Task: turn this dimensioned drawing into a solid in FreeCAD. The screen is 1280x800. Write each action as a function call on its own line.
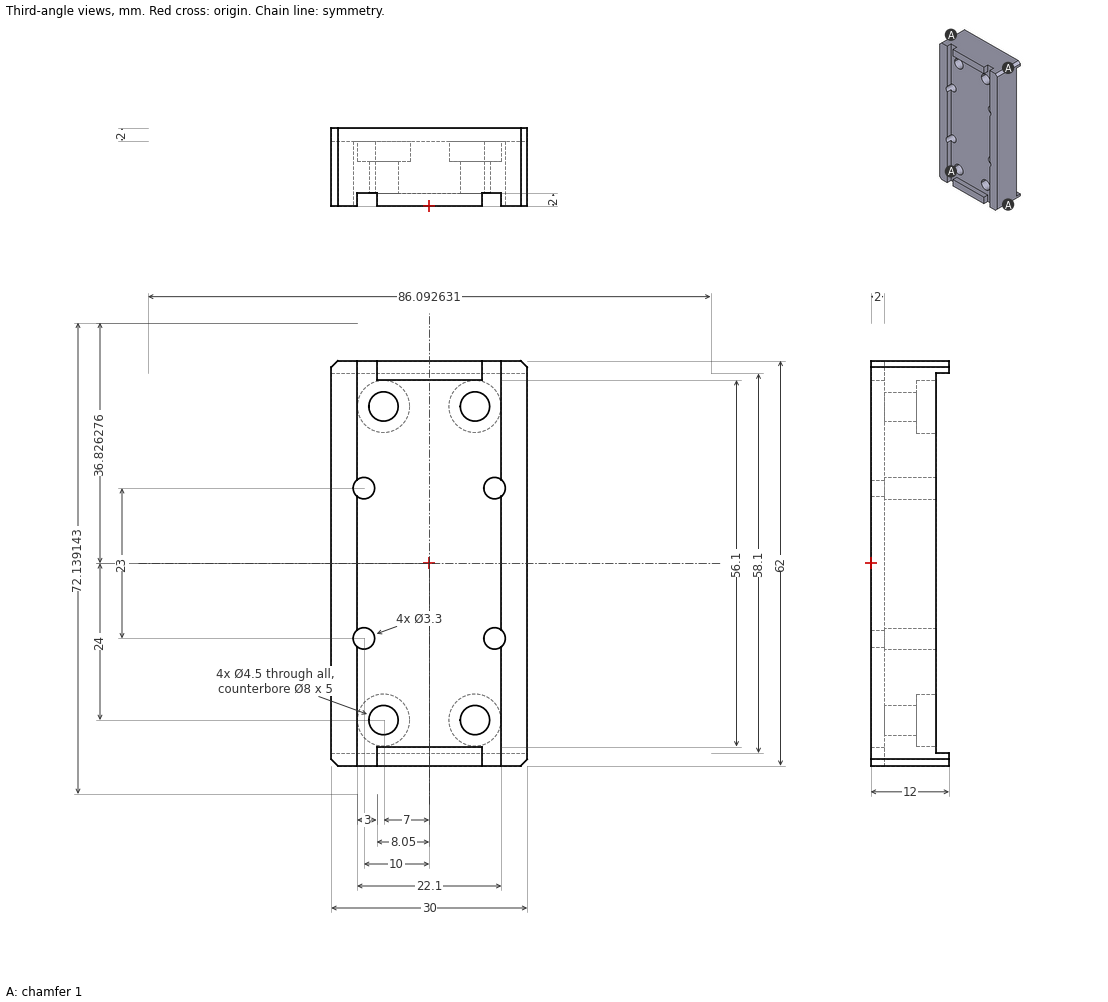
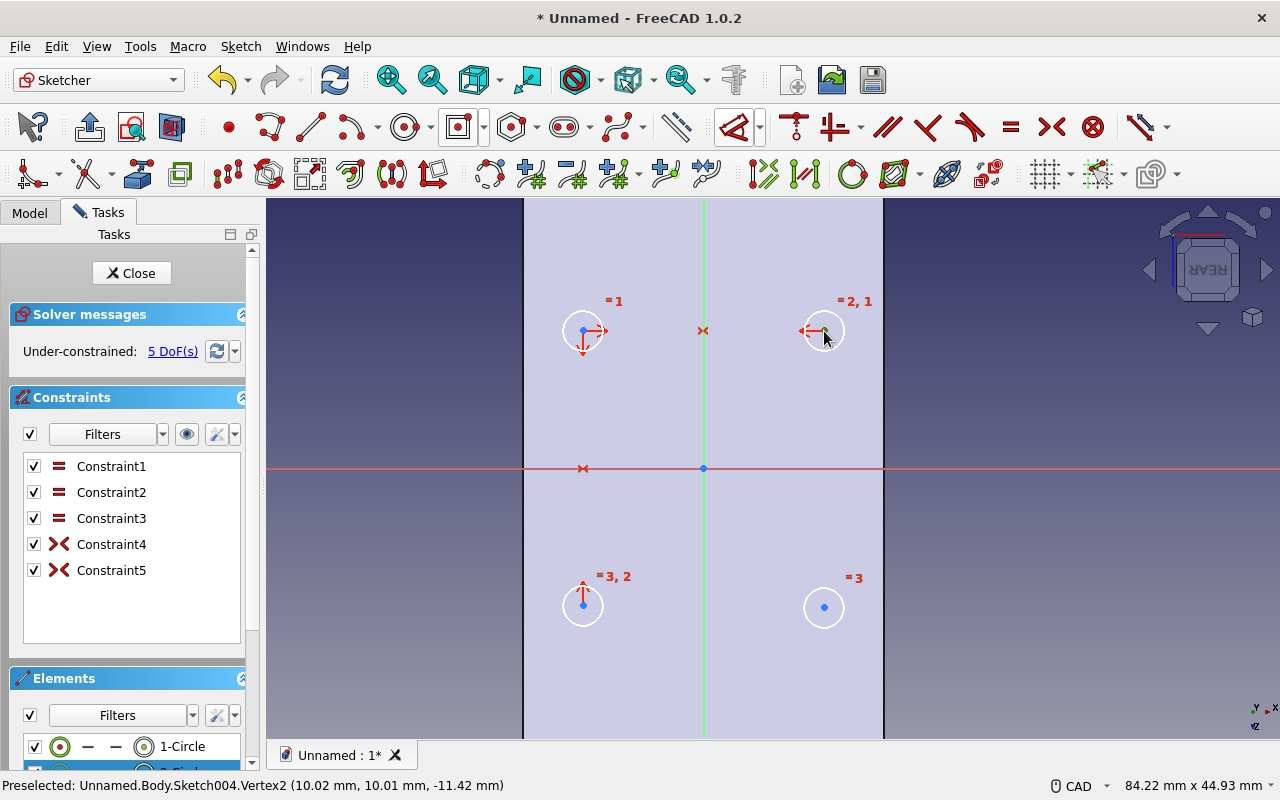
click(824, 608)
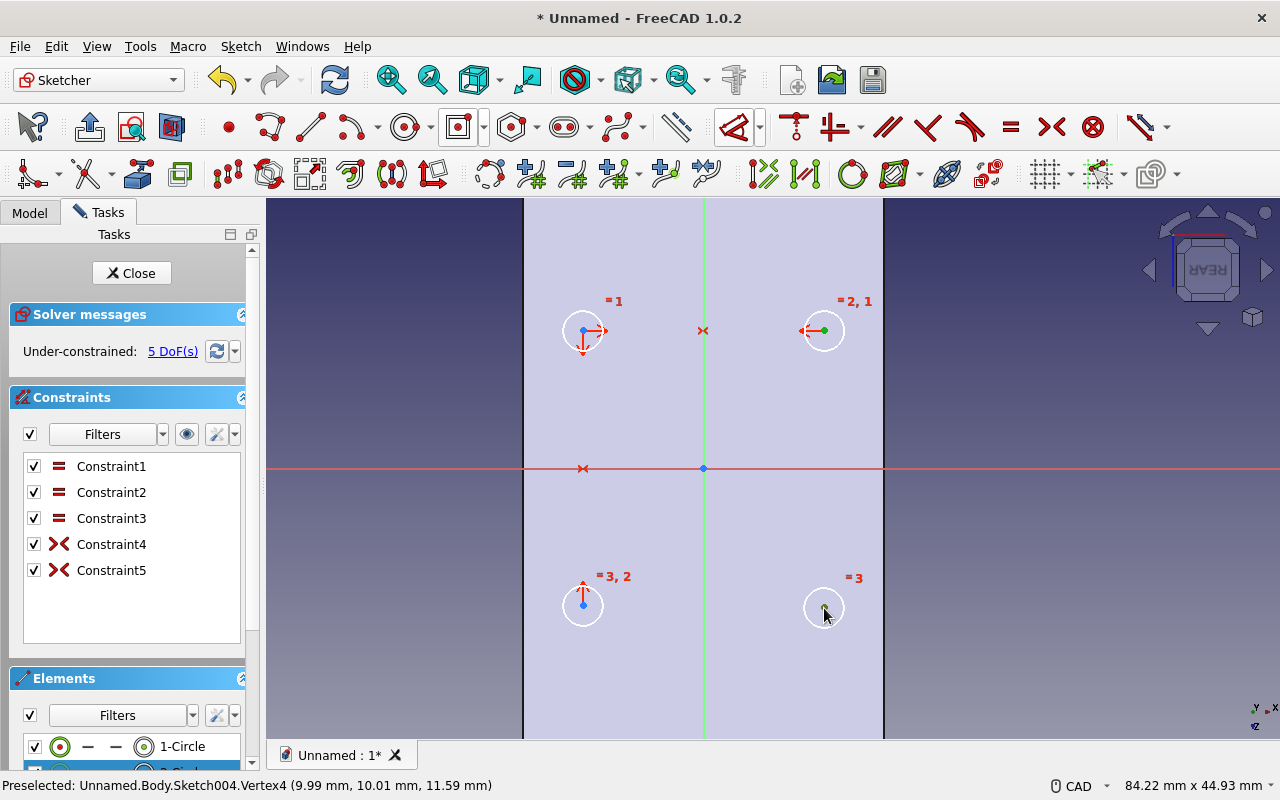
click(353, 468)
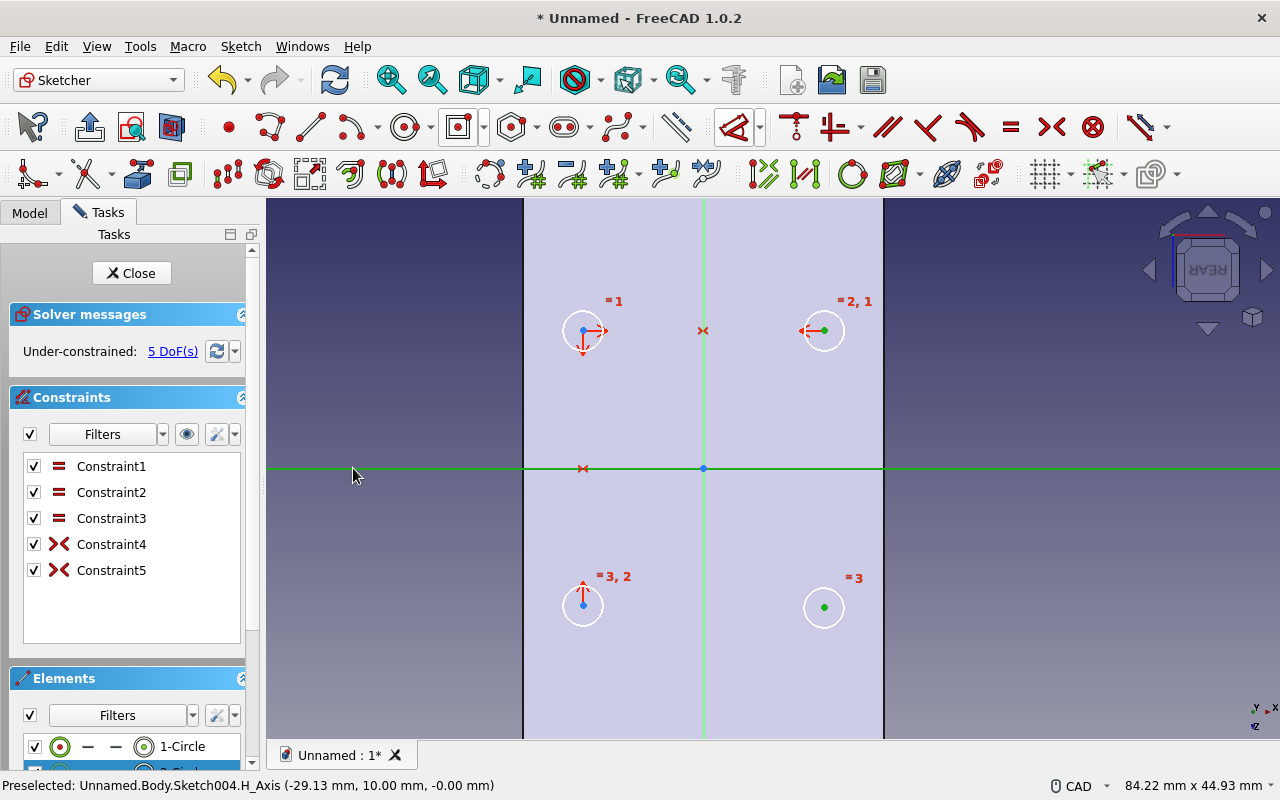
click(1052, 128)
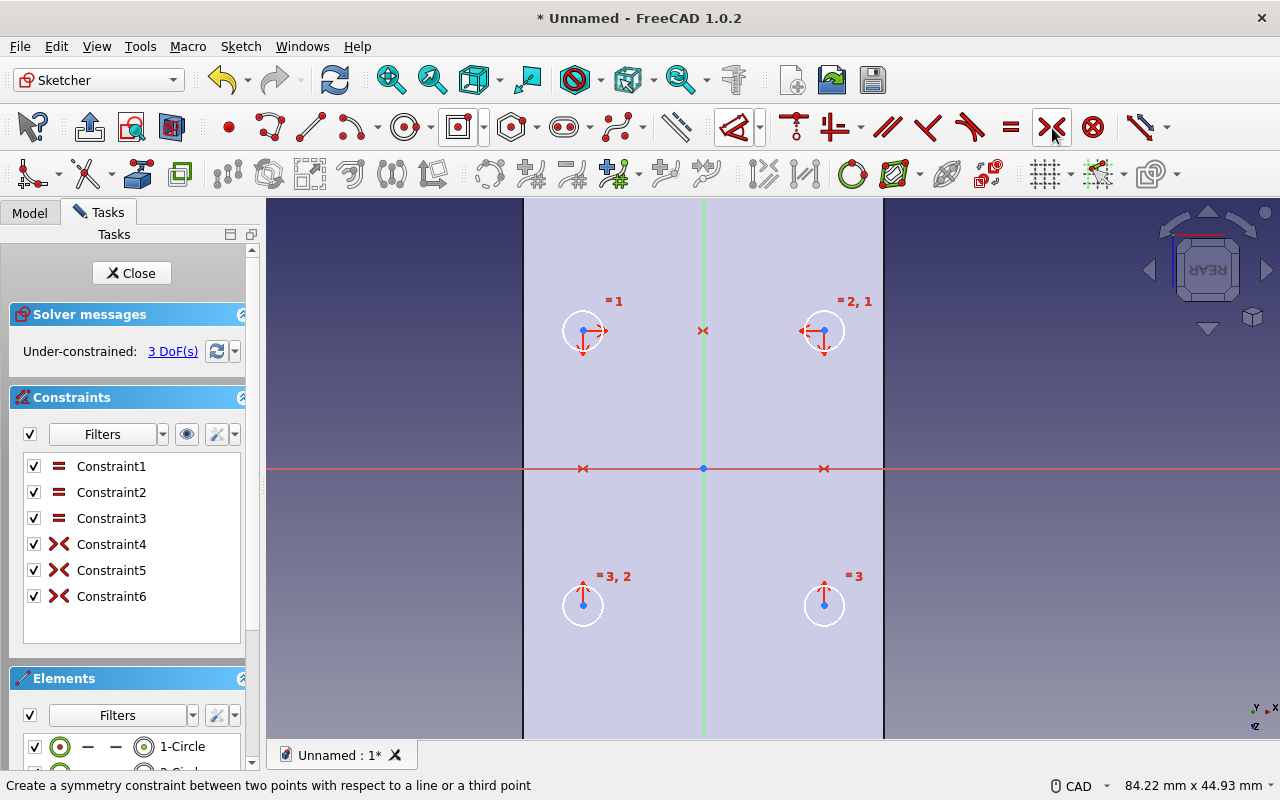
click(597, 317)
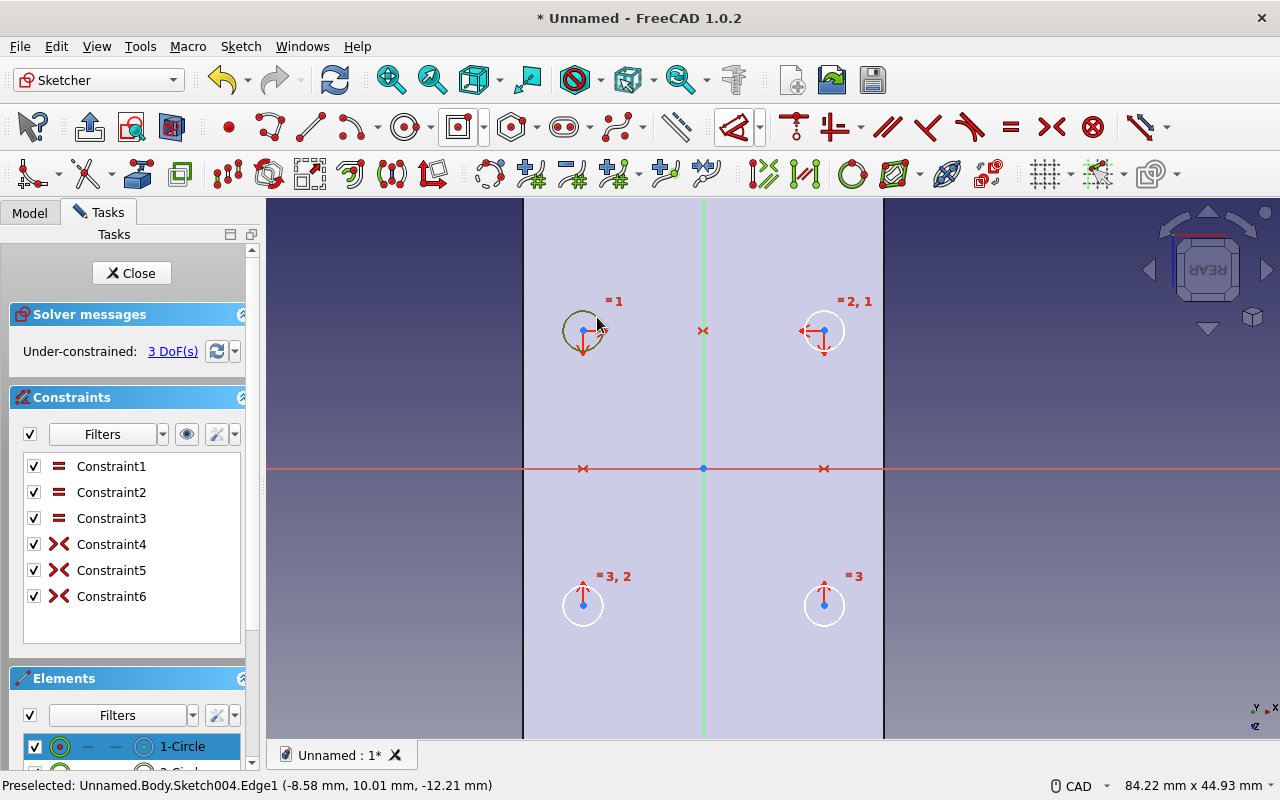
key(k)
key(o)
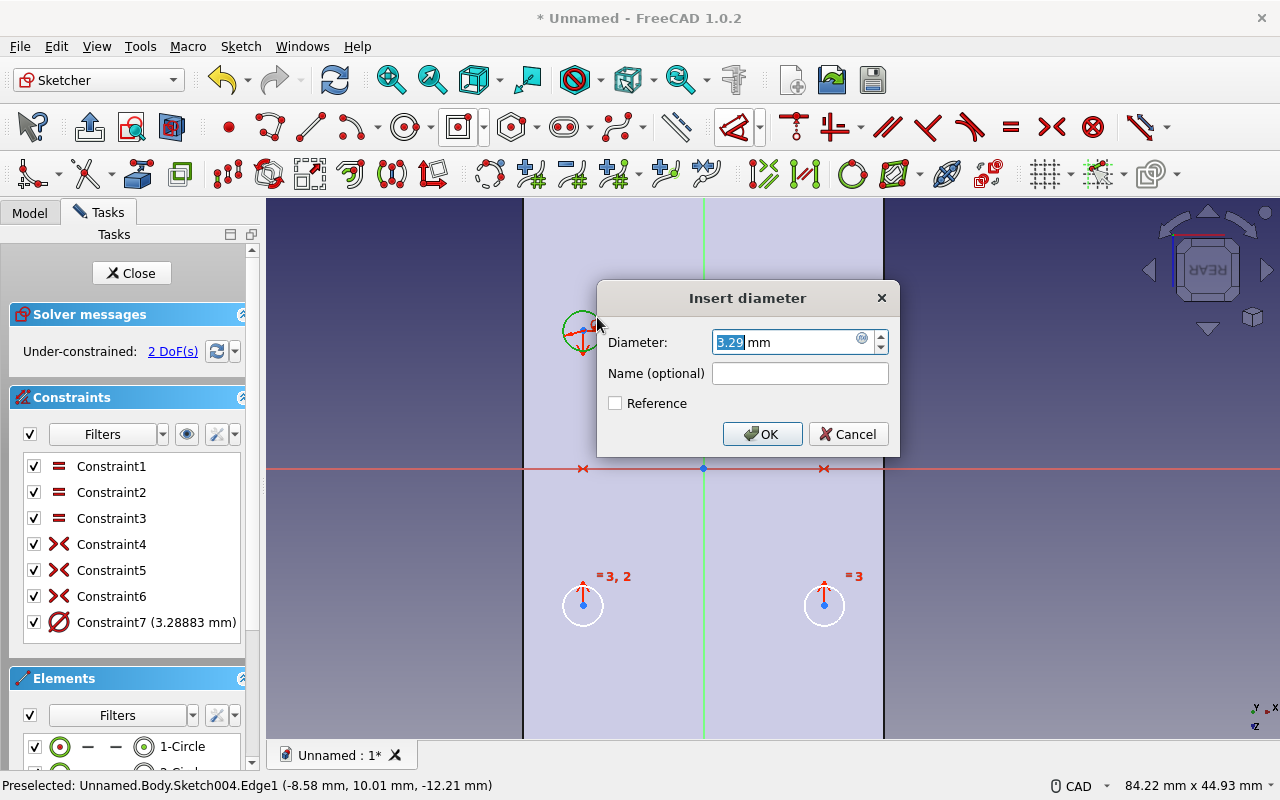
text(3.3)
key(Return)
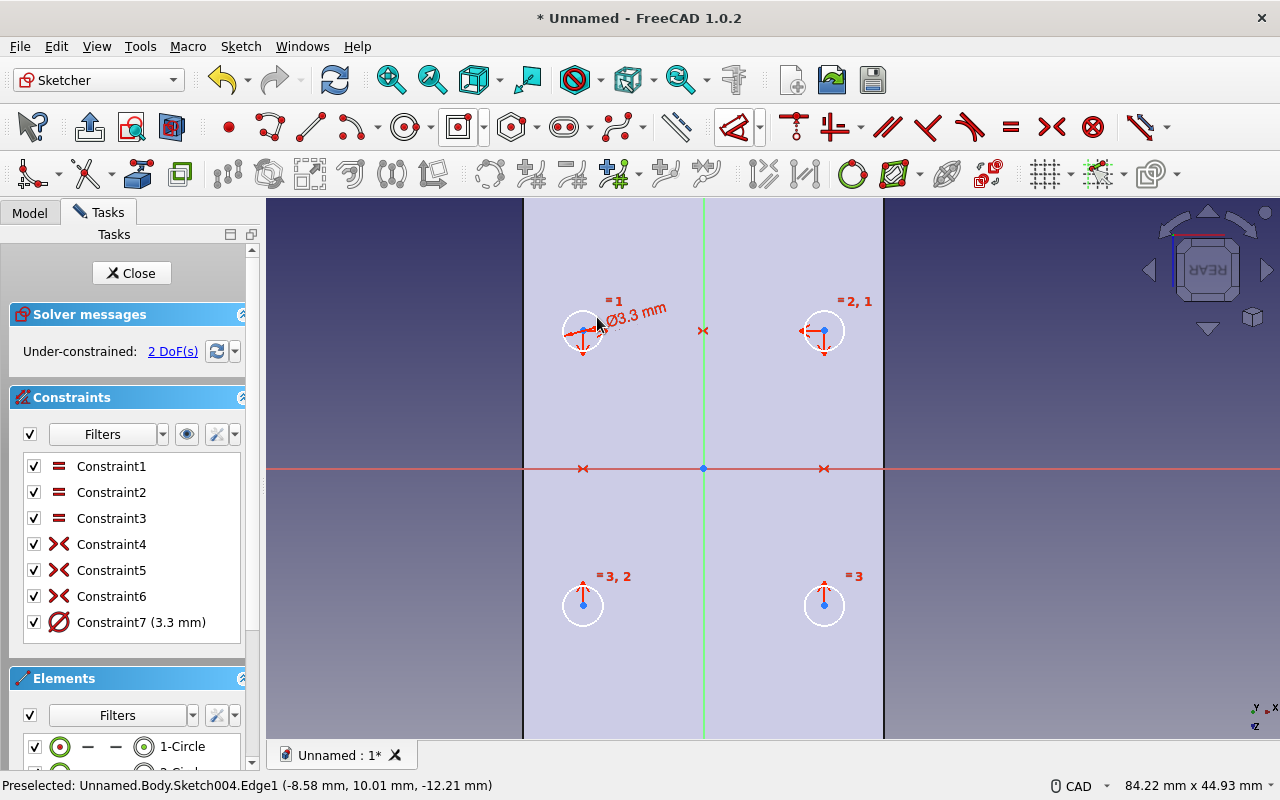
click(583, 331)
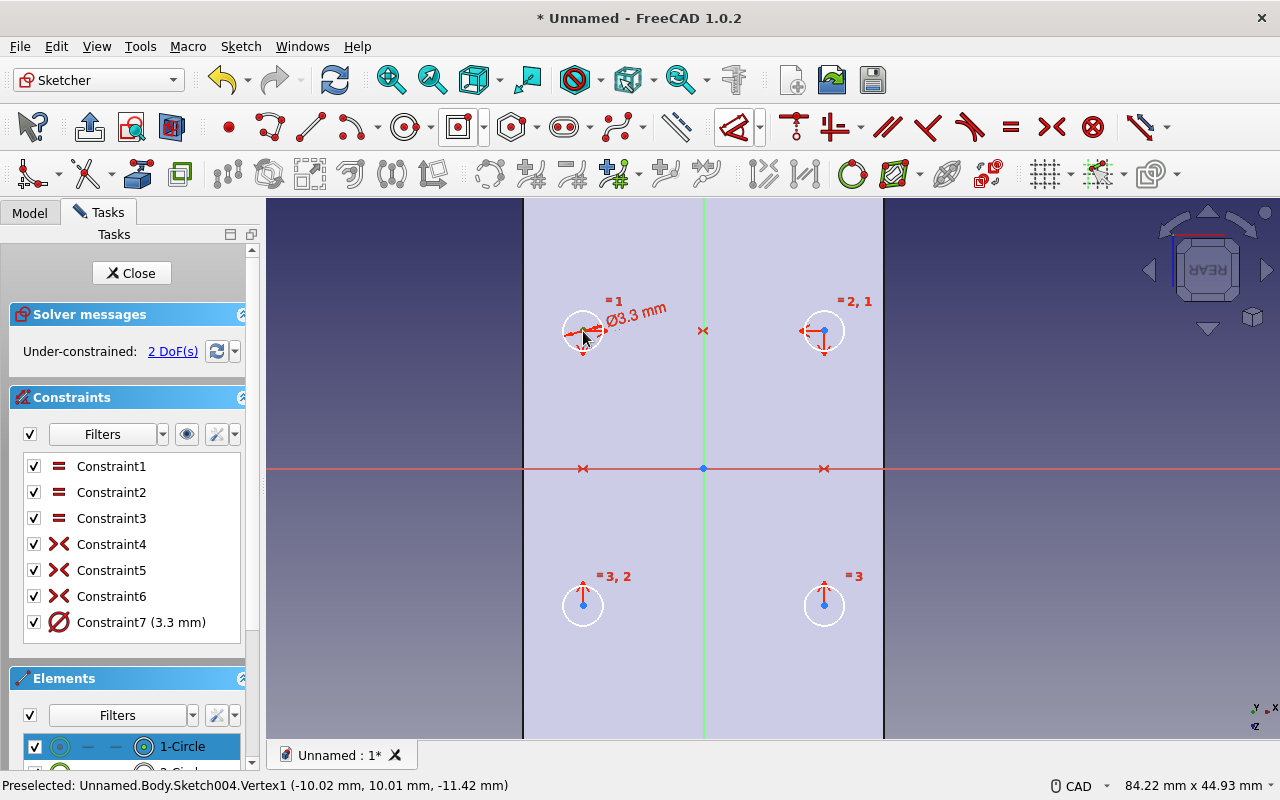
click(760, 128)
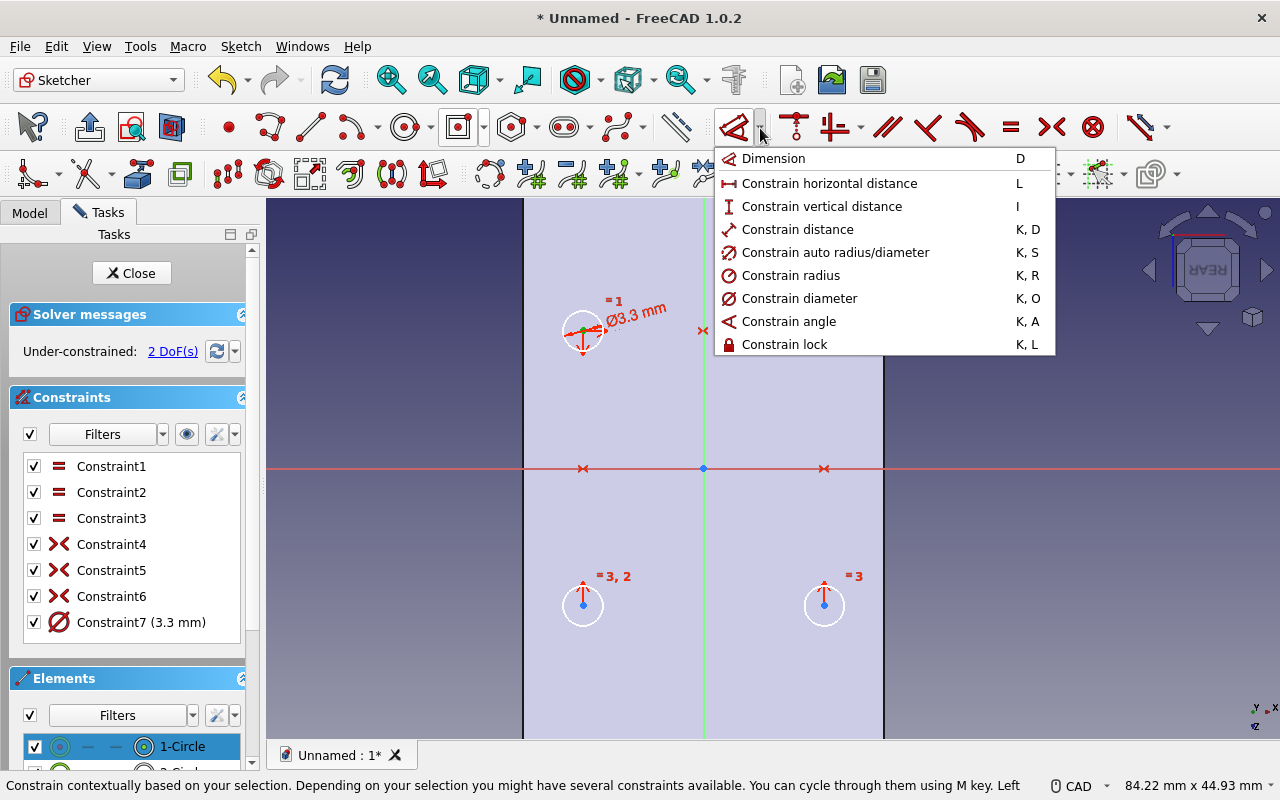
click(885, 184)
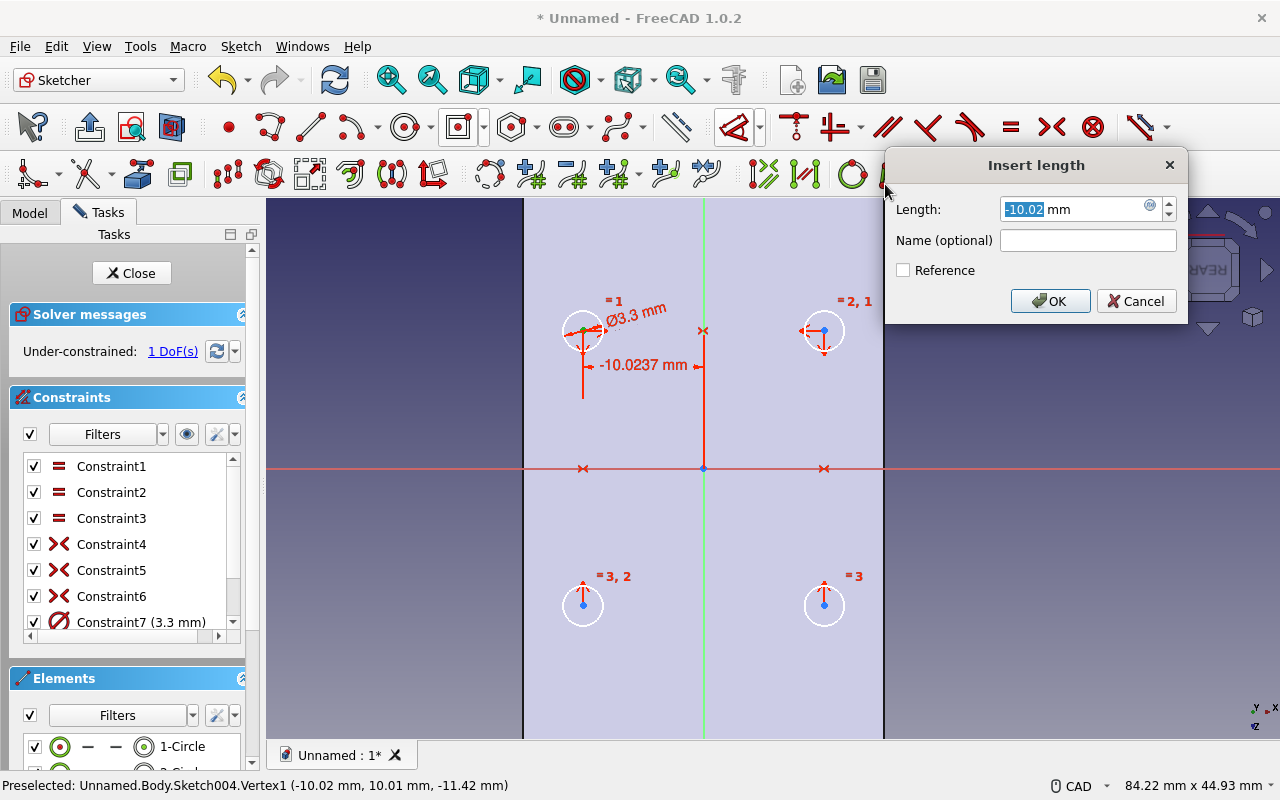
text(-10)
key(Return)